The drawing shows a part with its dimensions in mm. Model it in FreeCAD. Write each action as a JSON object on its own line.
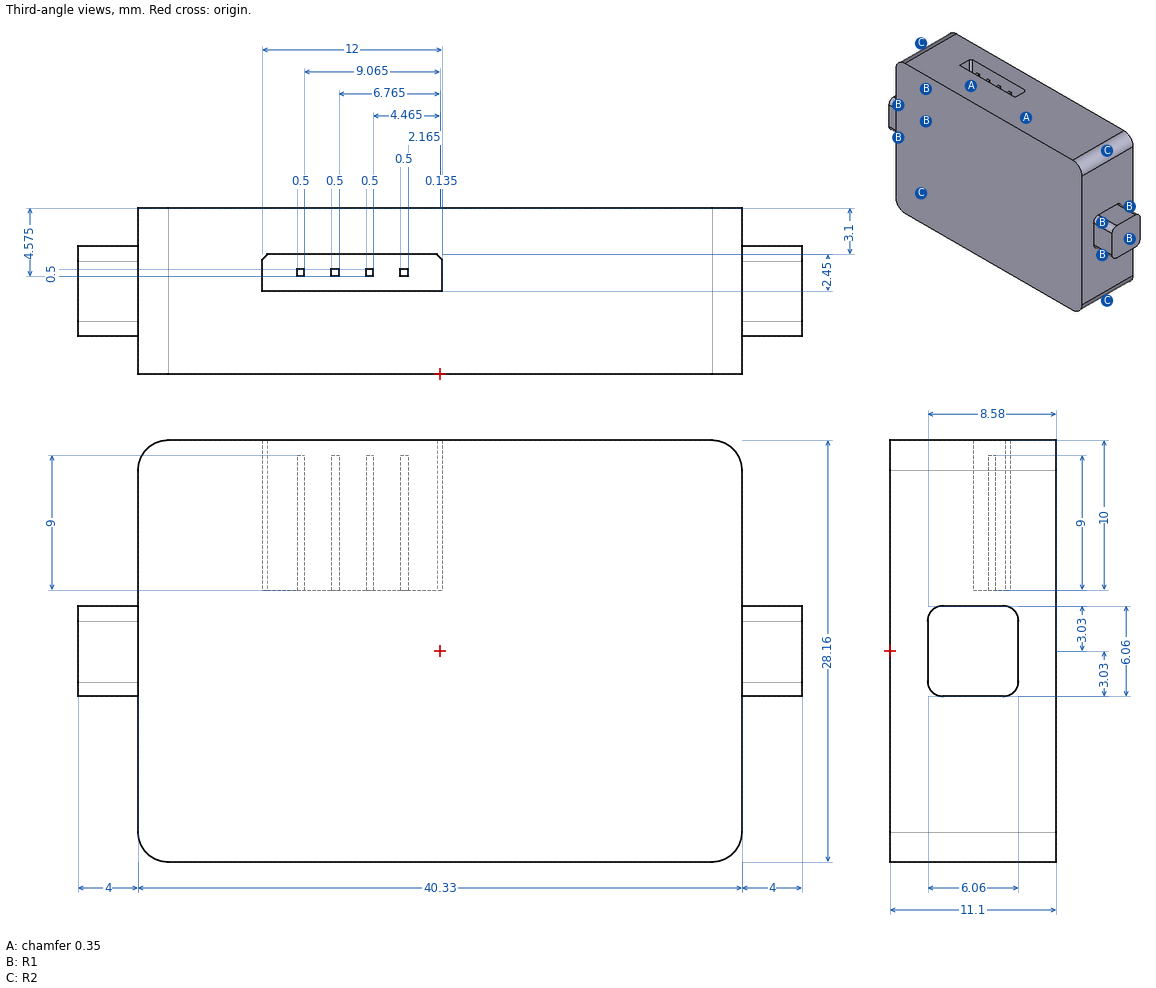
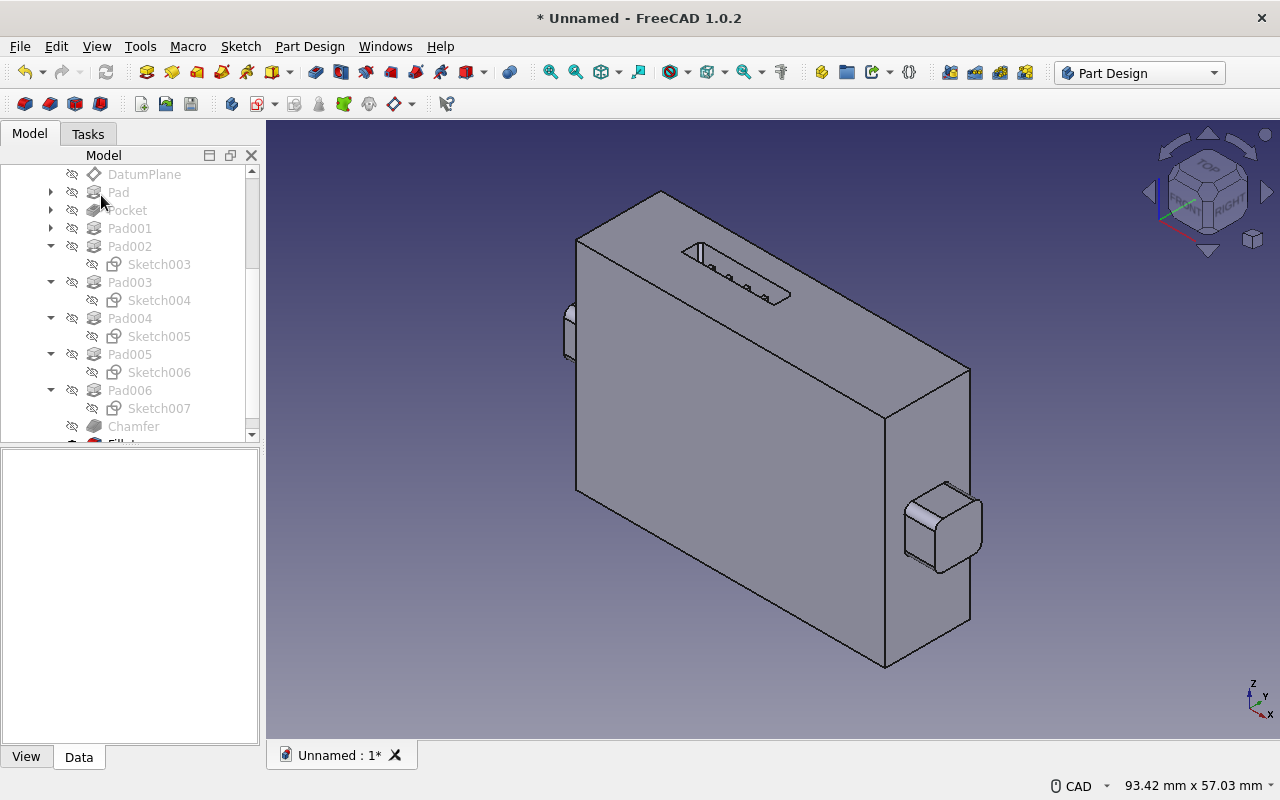
{"action": "left_click", "coordinate": [928, 393]}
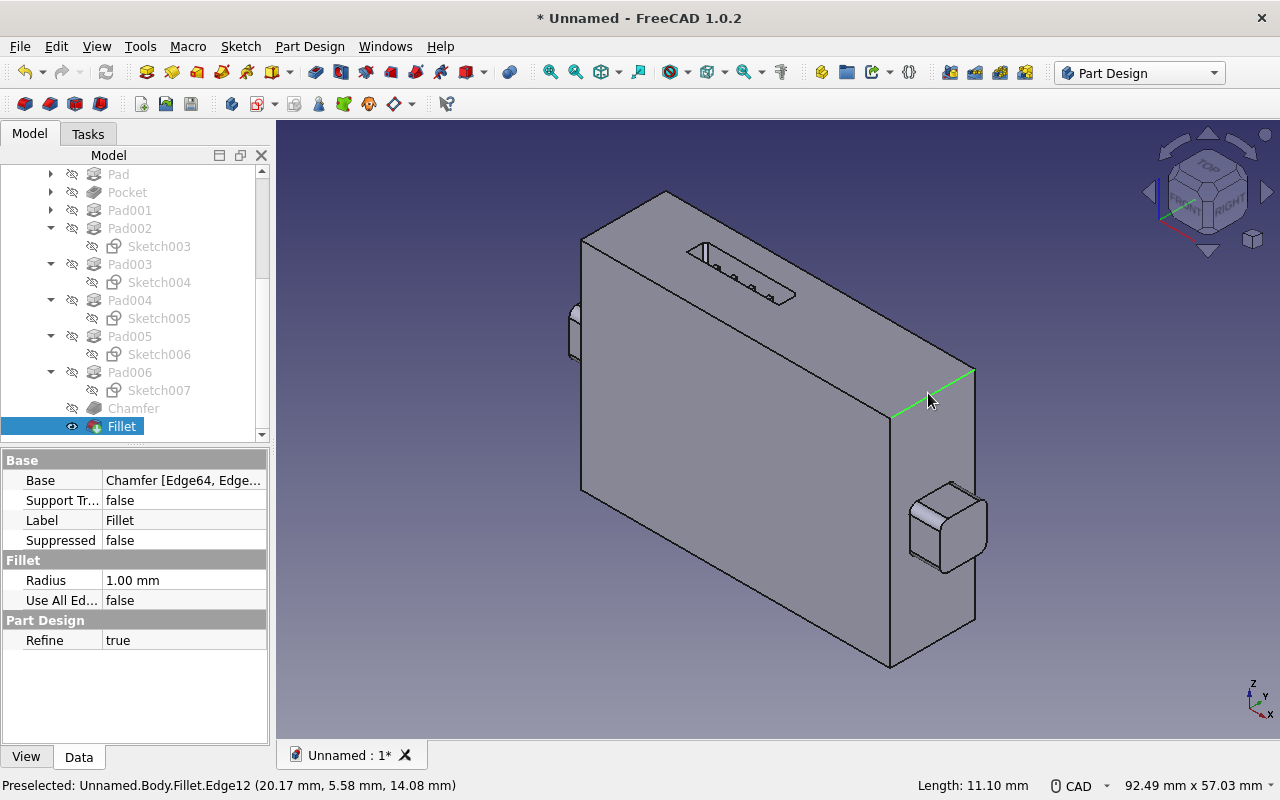
{"action": "key", "text": "2"}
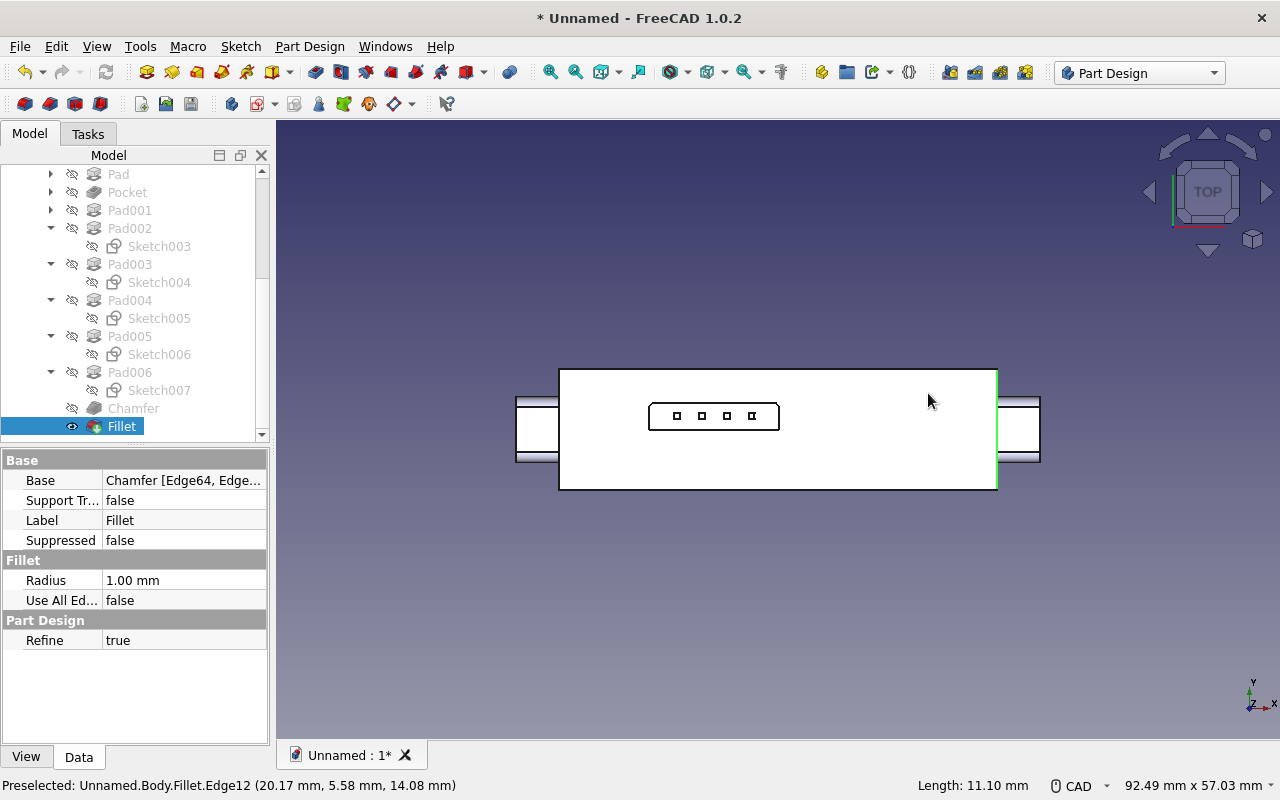
{"action": "left_click", "coordinate": [559, 428], "text": "ctrl"}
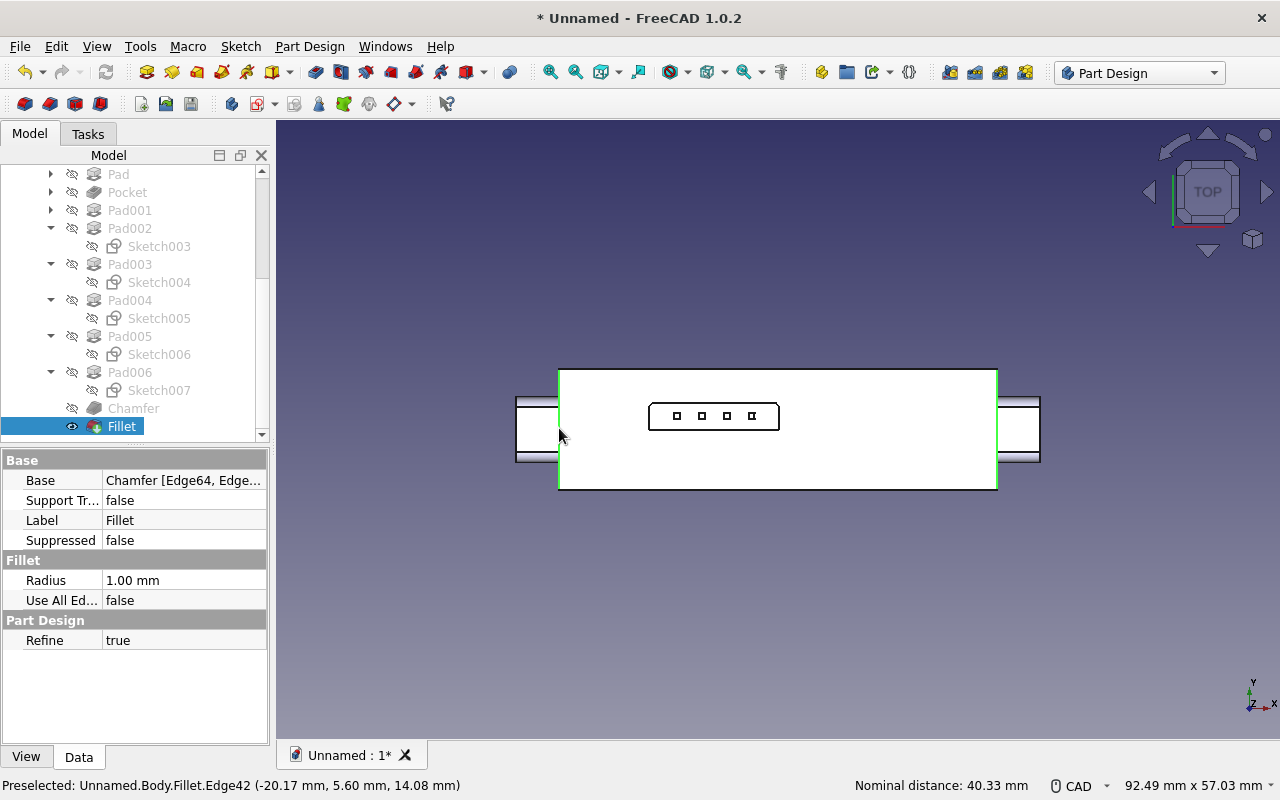
{"action": "key", "text": "1"}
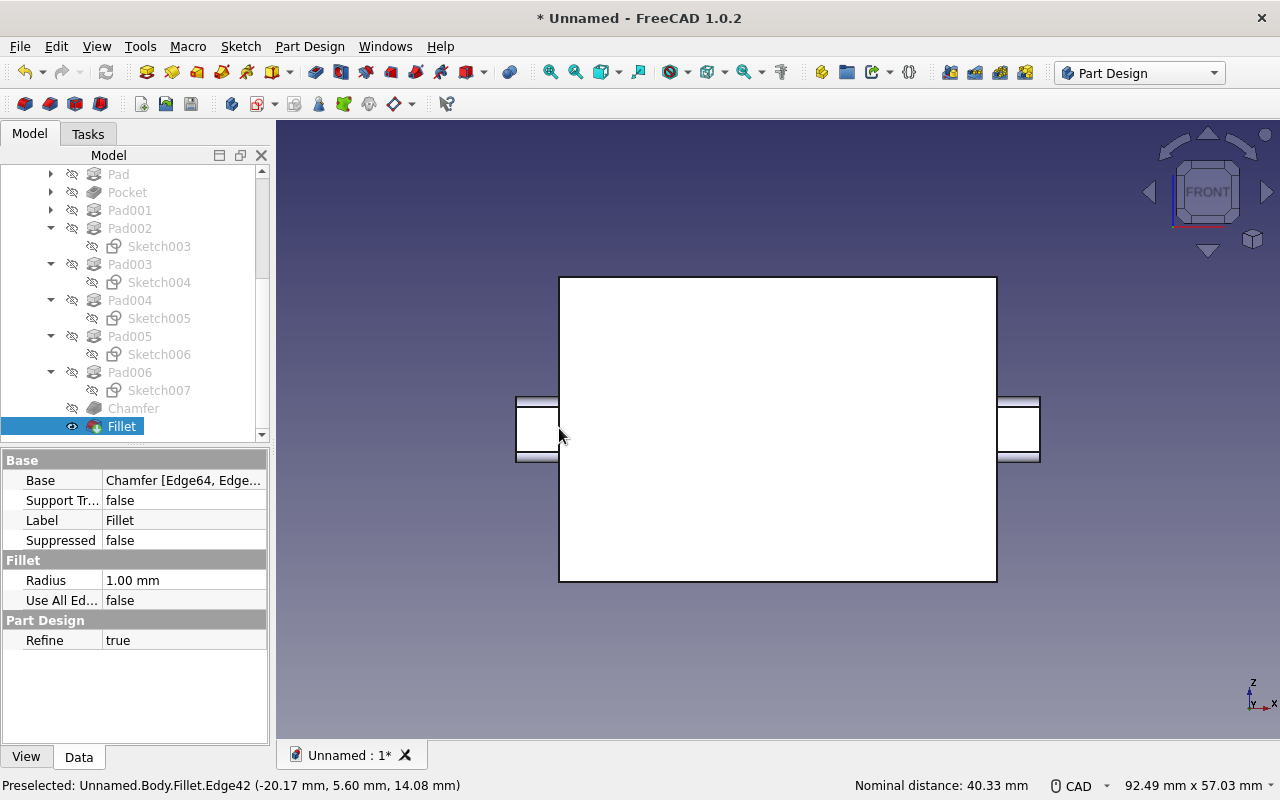
{"action": "key", "text": "3"}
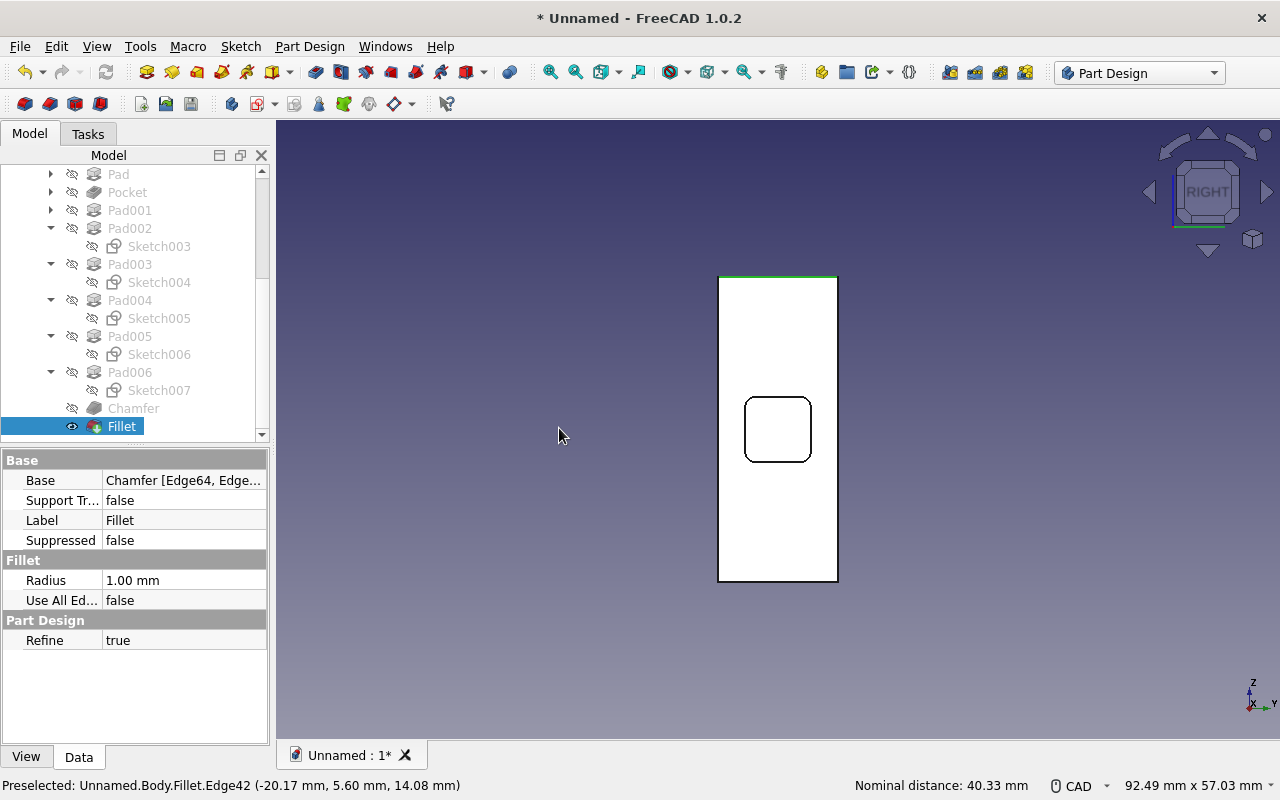
{"action": "left_click", "coordinate": [778, 581], "text": "ctrl"}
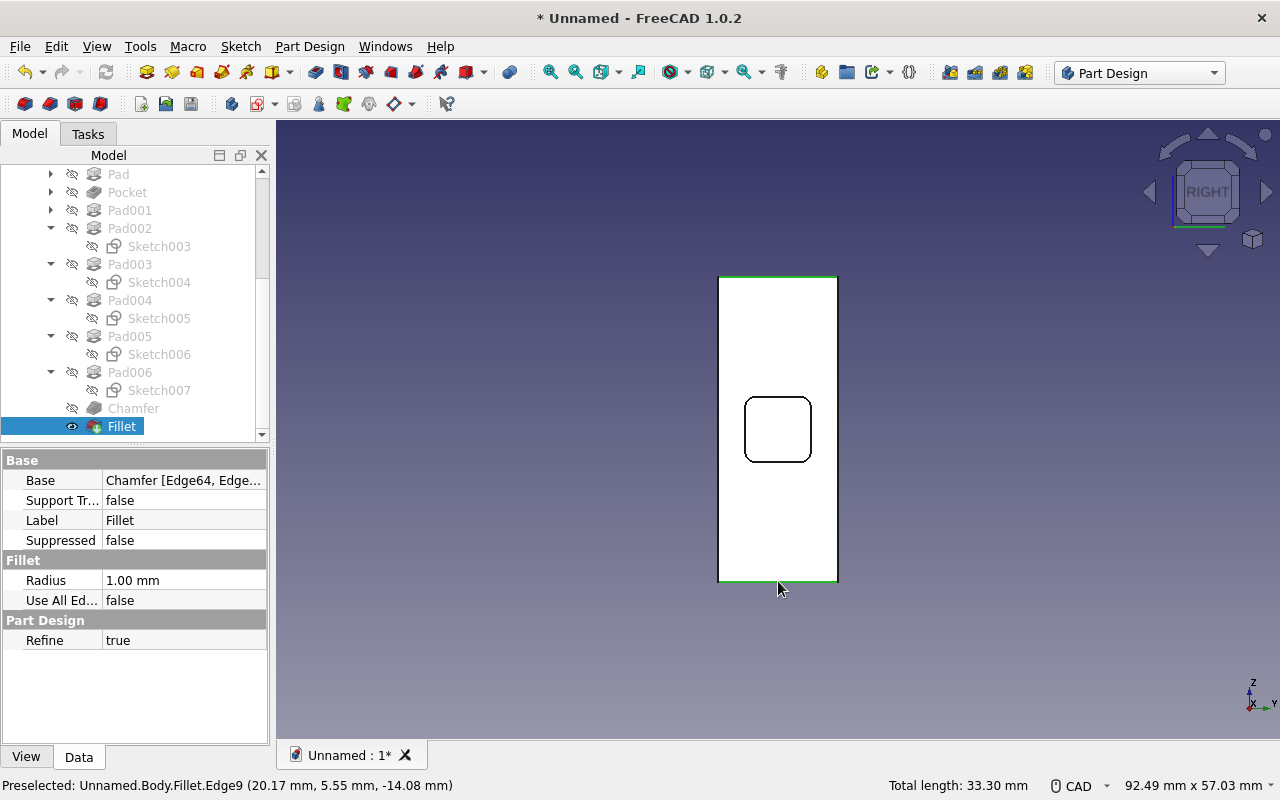
{"action": "key", "text": "5"}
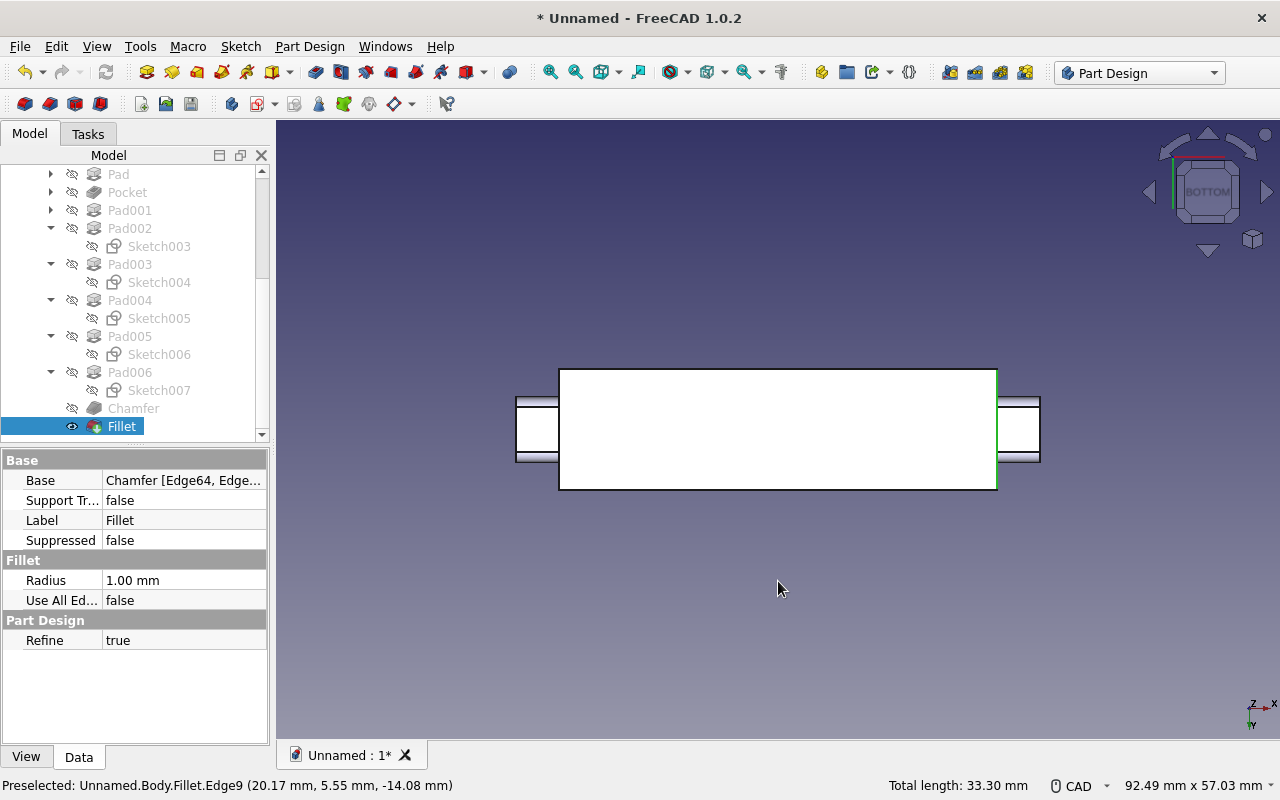
{"action": "left_click", "coordinate": [559, 429], "text": "ctrl"}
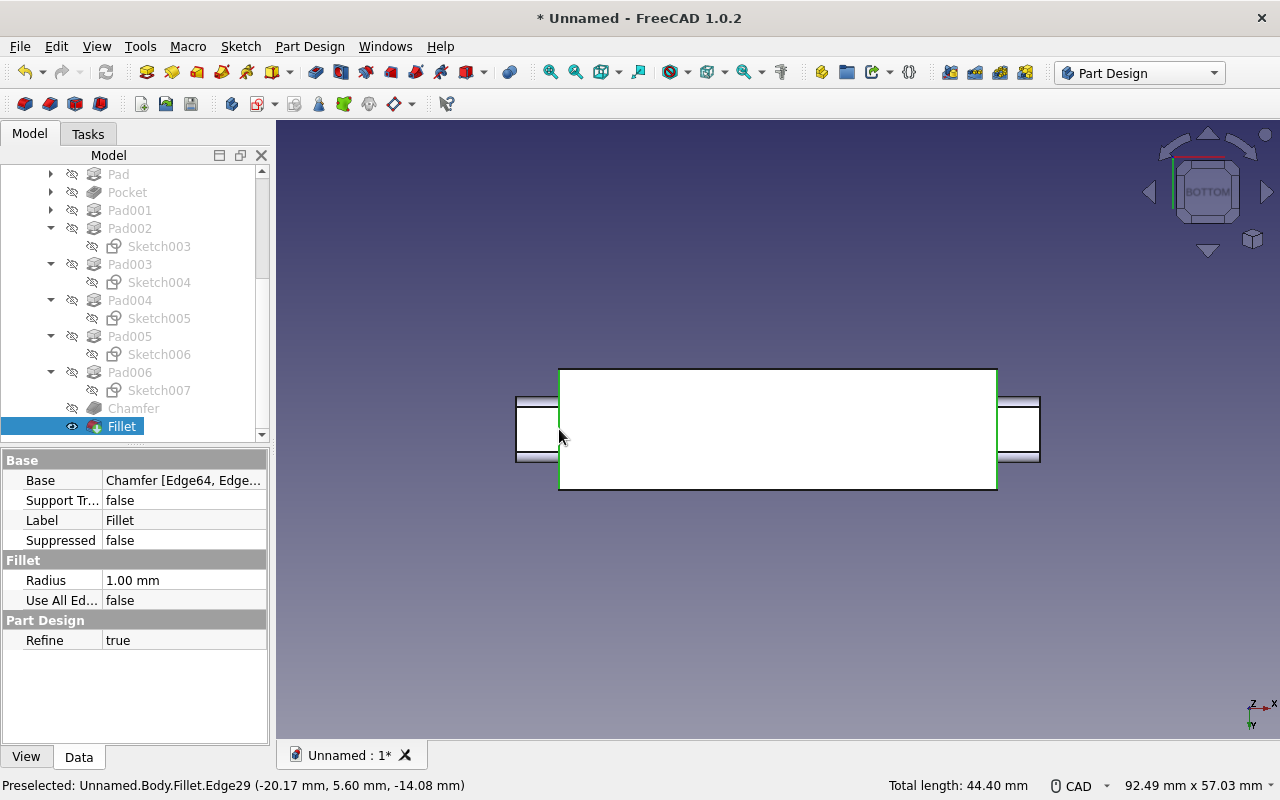
{"action": "left_click", "coordinate": [25, 104]}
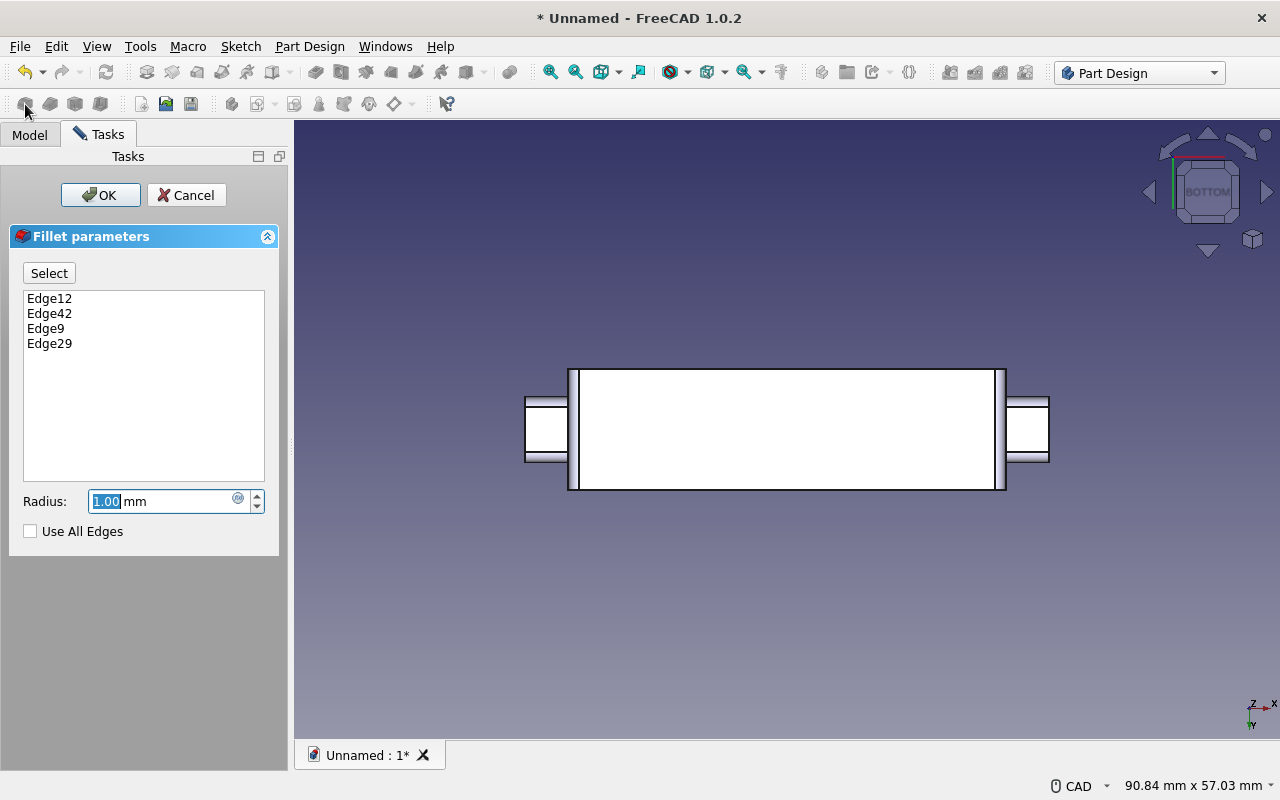
{"action": "type", "text": "2"}
{"action": "key", "text": "Tab"}